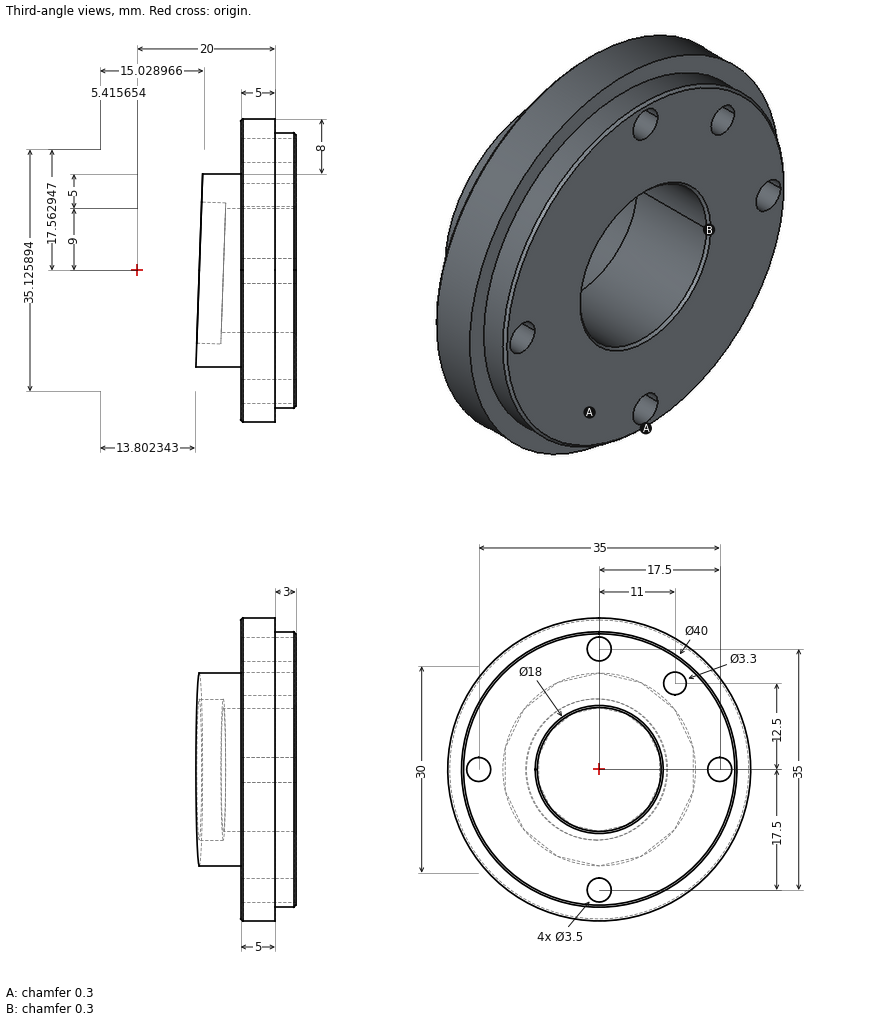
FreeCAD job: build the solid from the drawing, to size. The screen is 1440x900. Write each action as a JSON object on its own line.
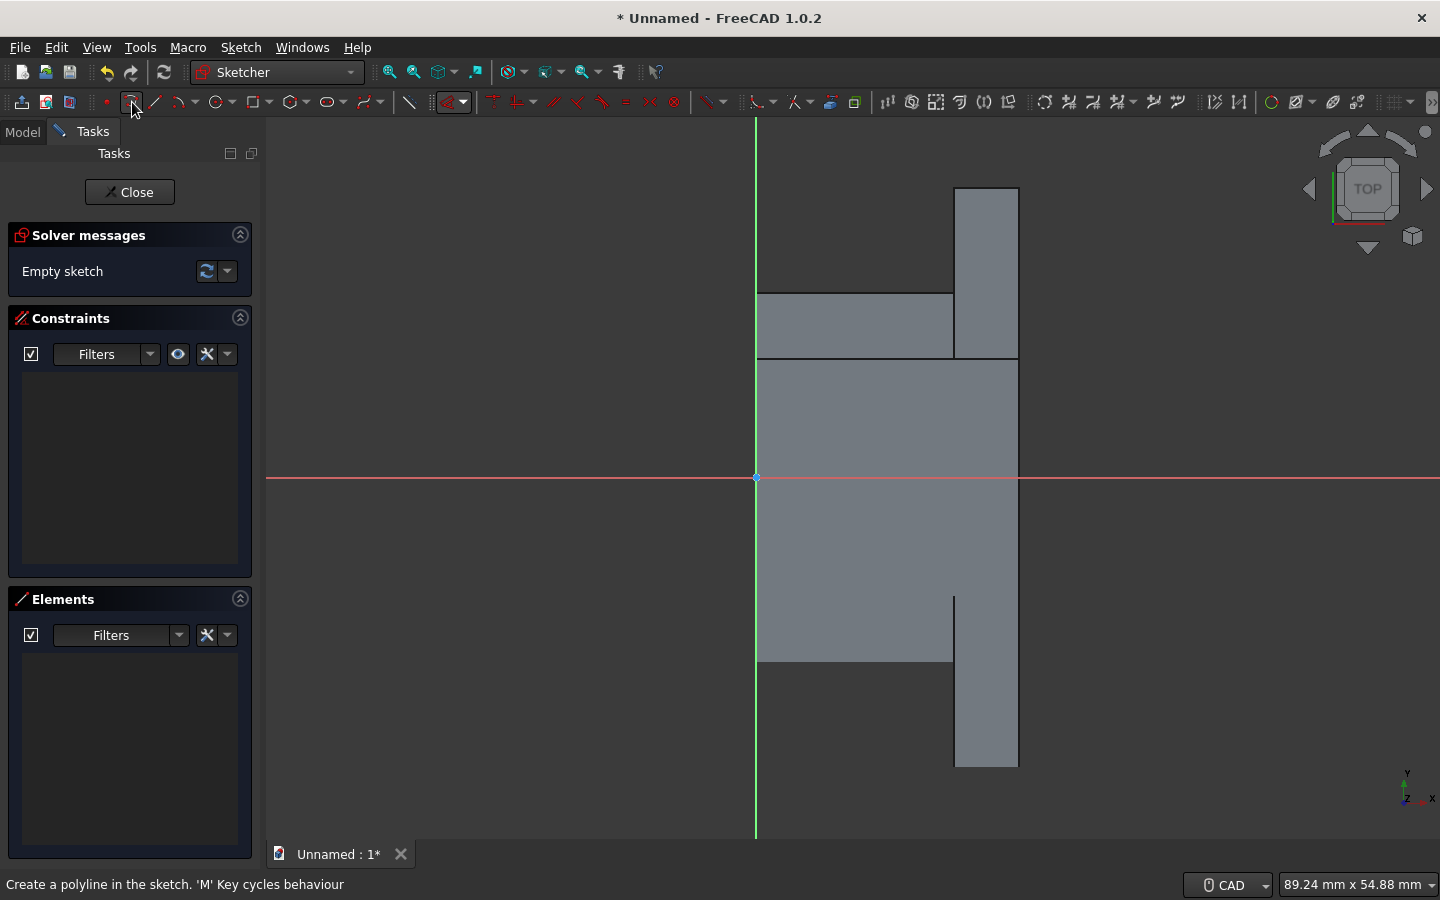
{"action": "left_click", "coordinate": [685, 247]}
{"action": "left_click", "coordinate": [685, 709]}
{"action": "left_click", "coordinate": [867, 709]}
{"action": "left_click", "coordinate": [889, 247]}
{"action": "left_click", "coordinate": [685, 248]}
{"action": "key", "text": "Escape"}
{"action": "key", "text": "Escape"}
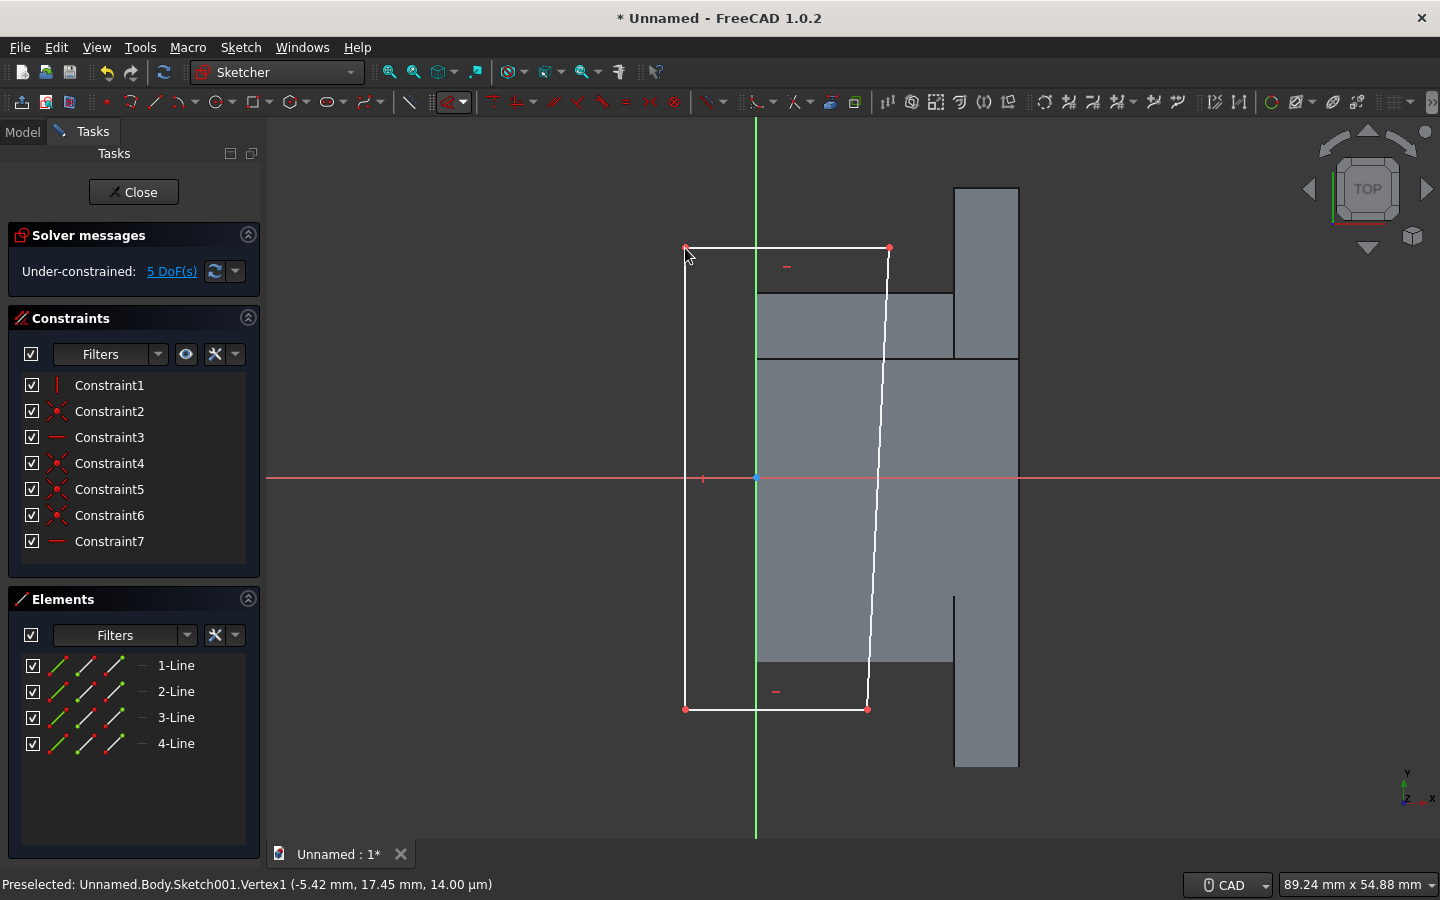
{"action": "left_click", "coordinate": [685, 387]}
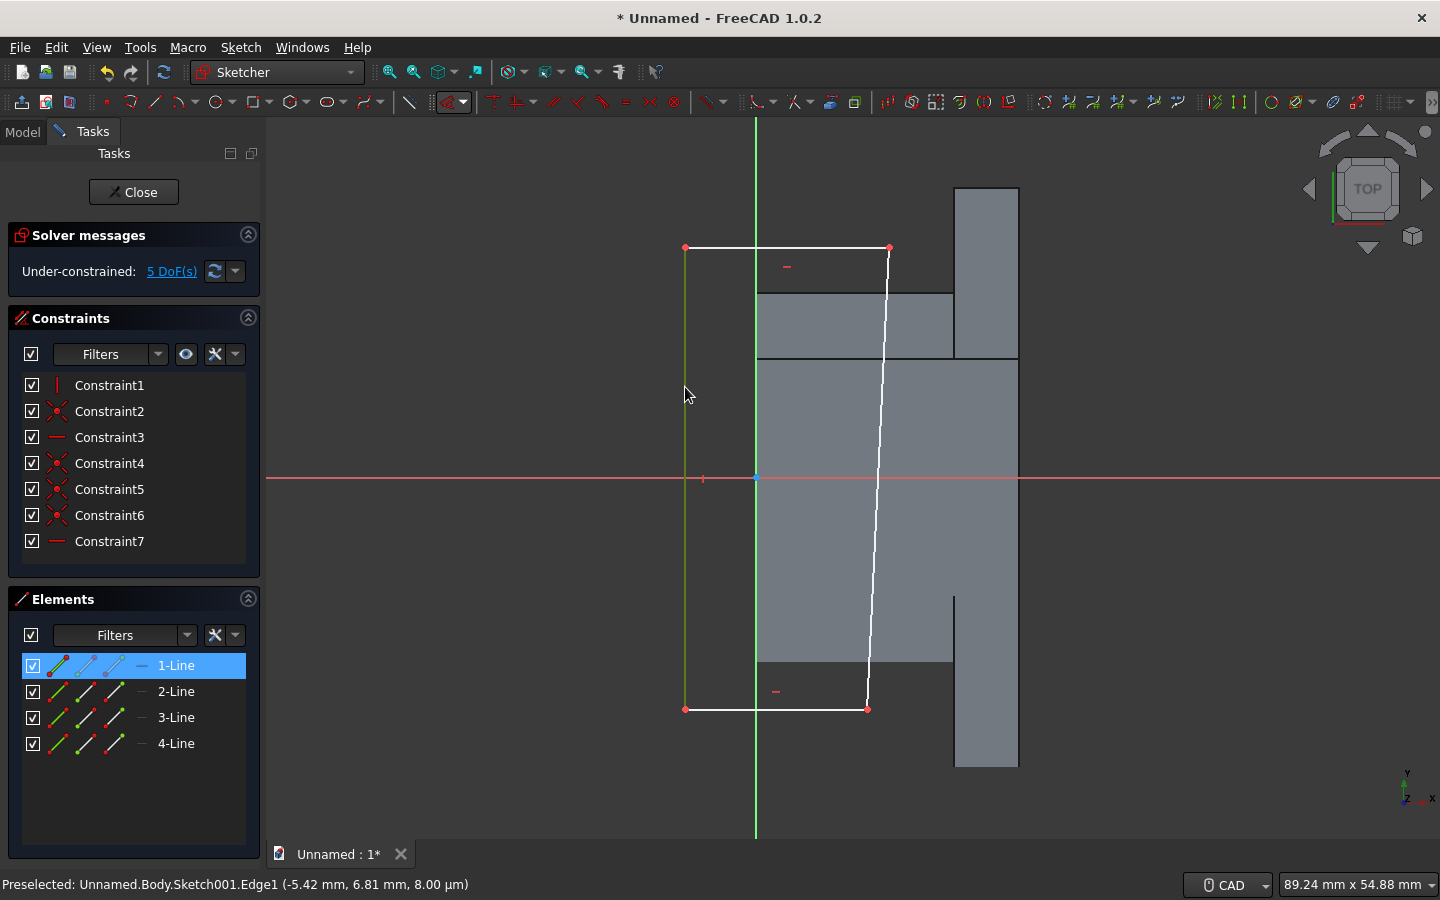
{"action": "left_click", "coordinate": [466, 102]}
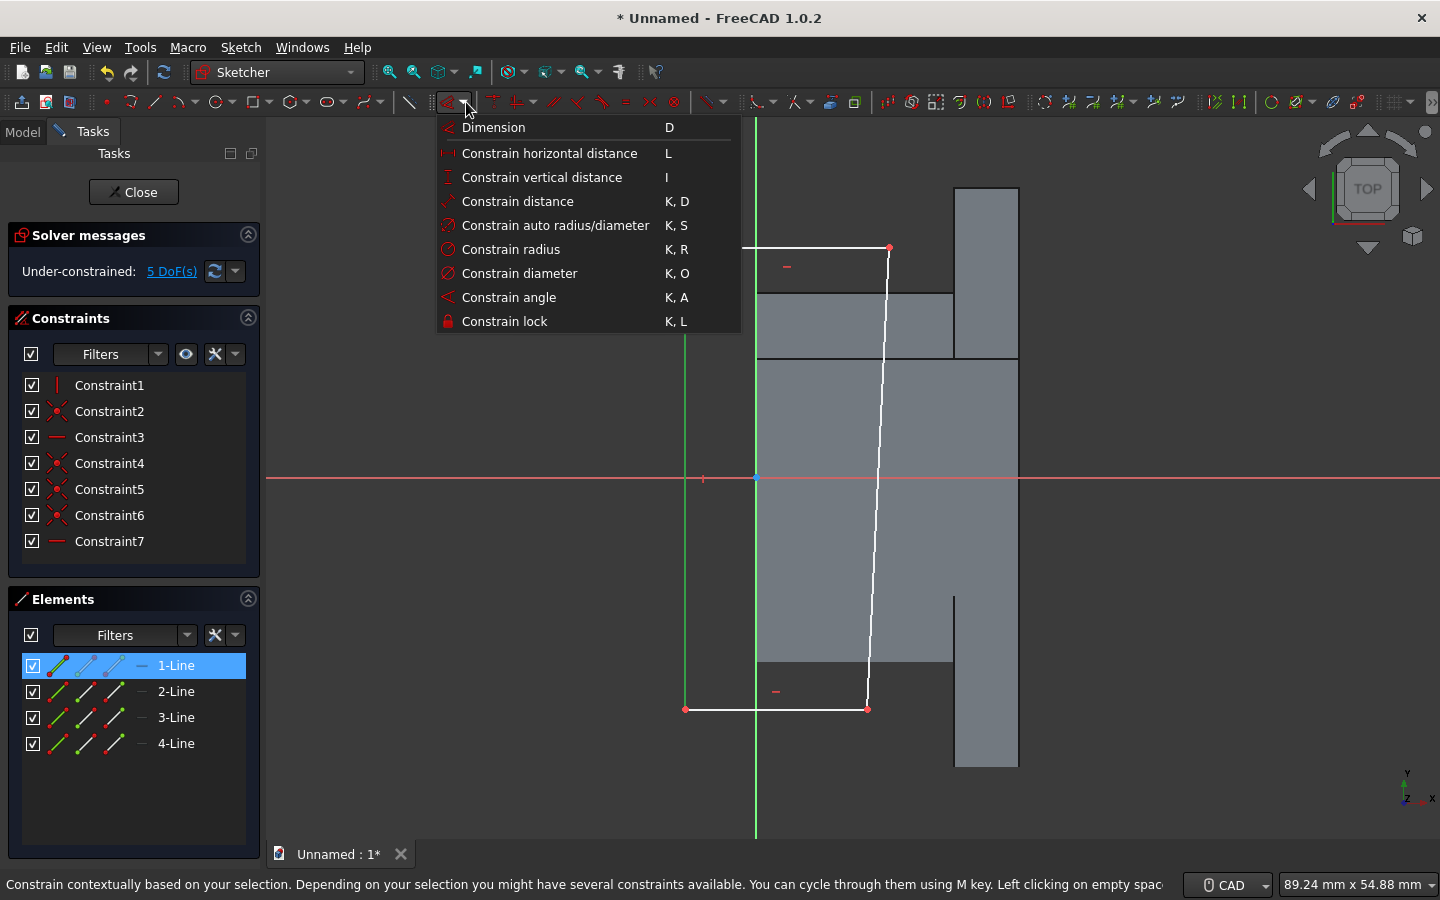
{"action": "left_click", "coordinate": [589, 177]}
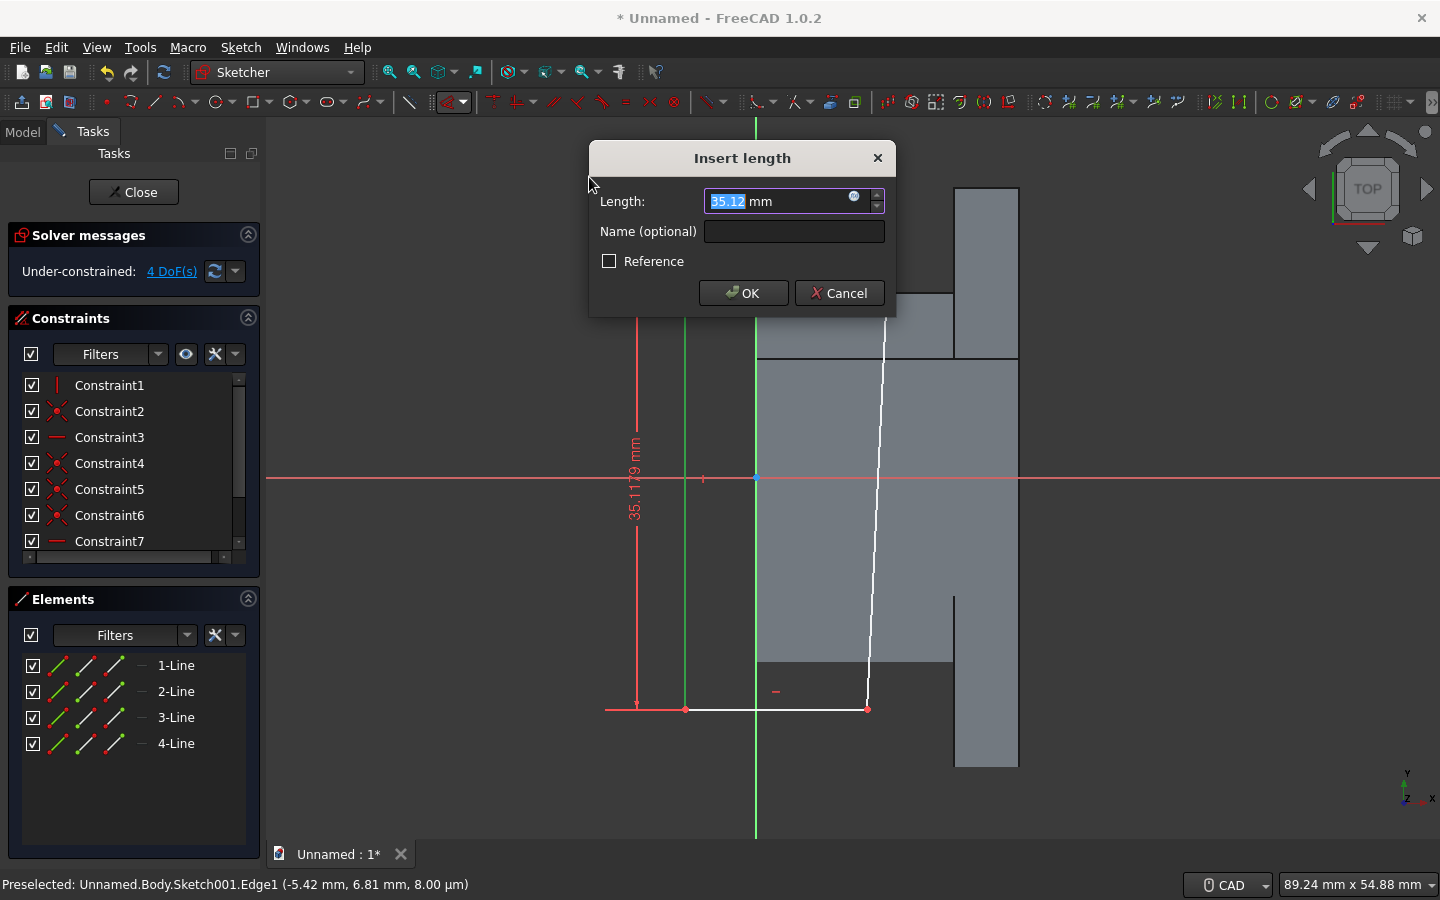
{"action": "type", "text": "35.125894"}
{"action": "key", "text": "Return"}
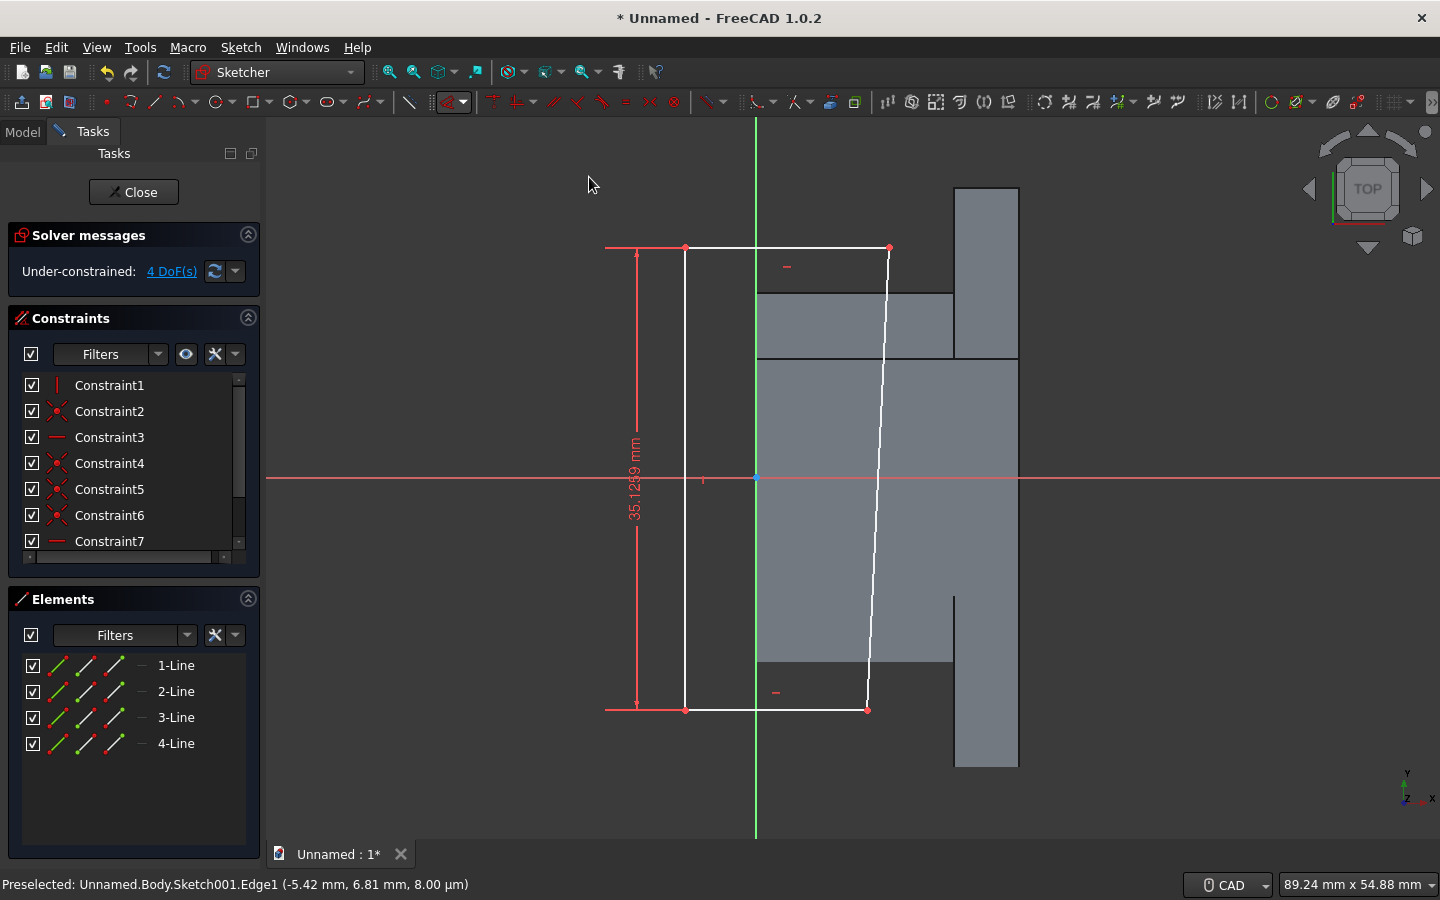
{"action": "left_click", "coordinate": [740, 710]}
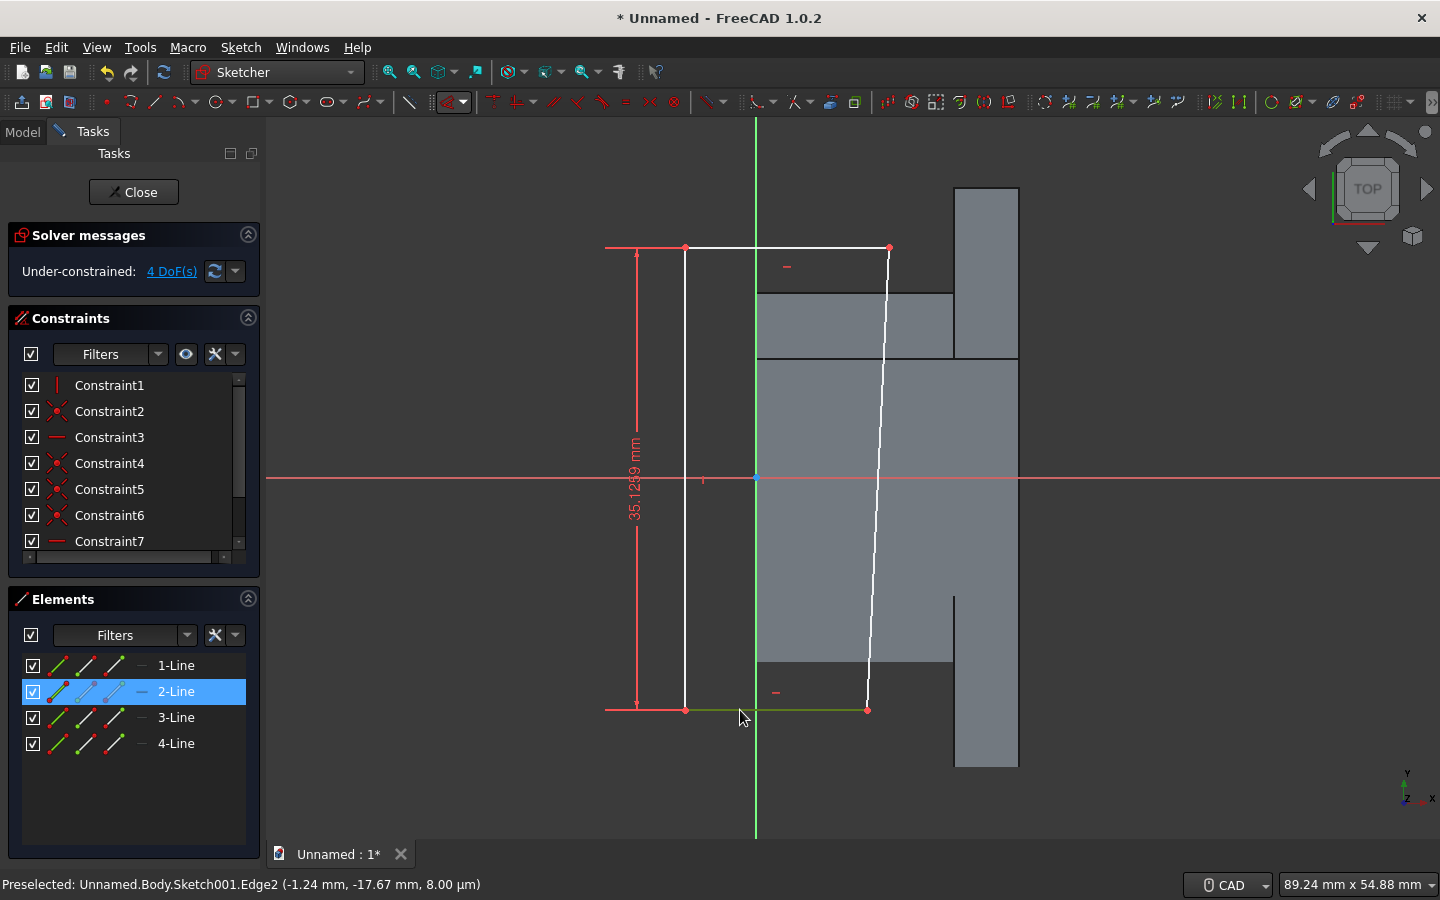
{"action": "left_click", "coordinate": [466, 102]}